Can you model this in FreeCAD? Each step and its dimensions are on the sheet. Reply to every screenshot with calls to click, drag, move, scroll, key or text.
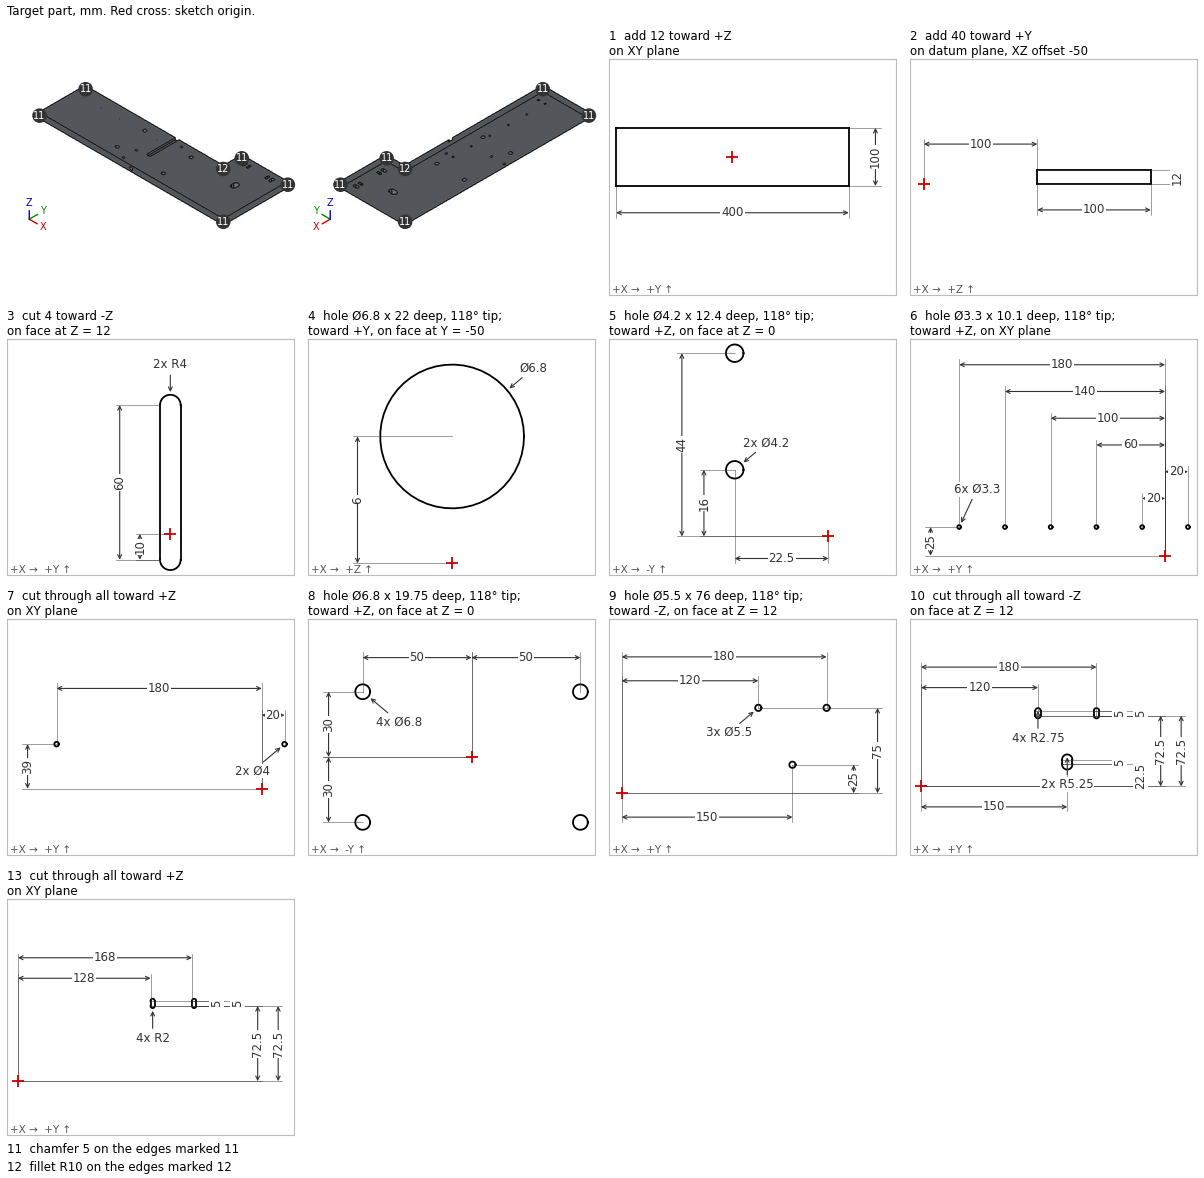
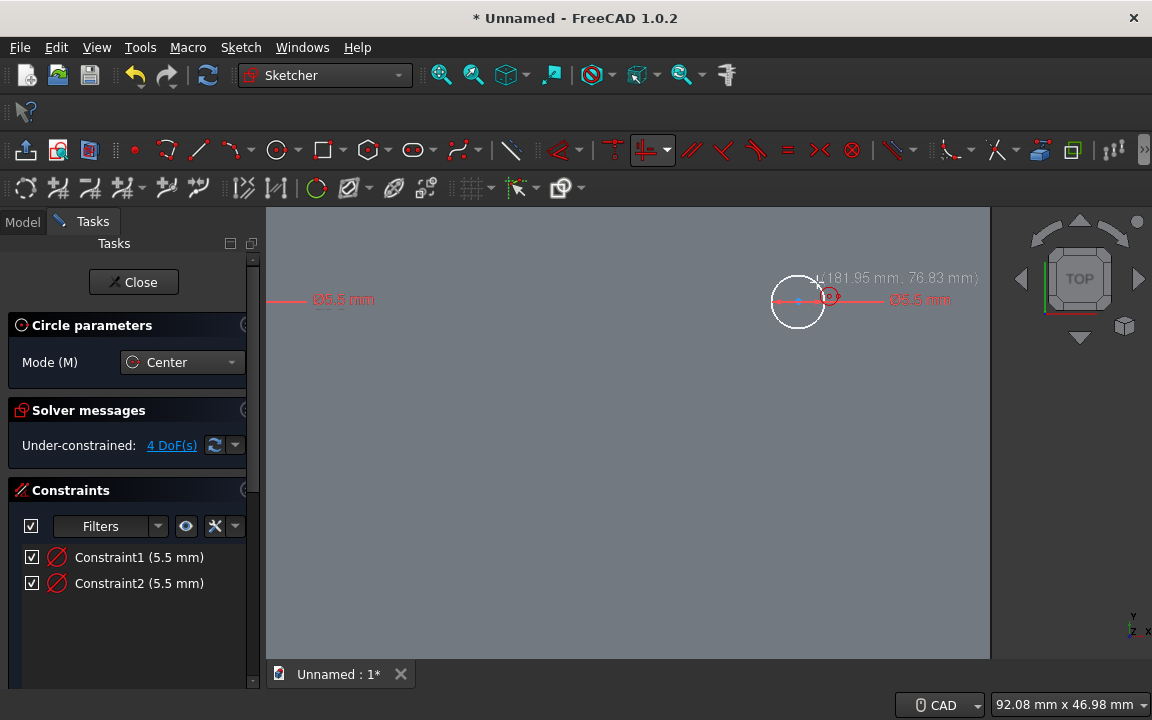
scroll(800, 301, down, 3)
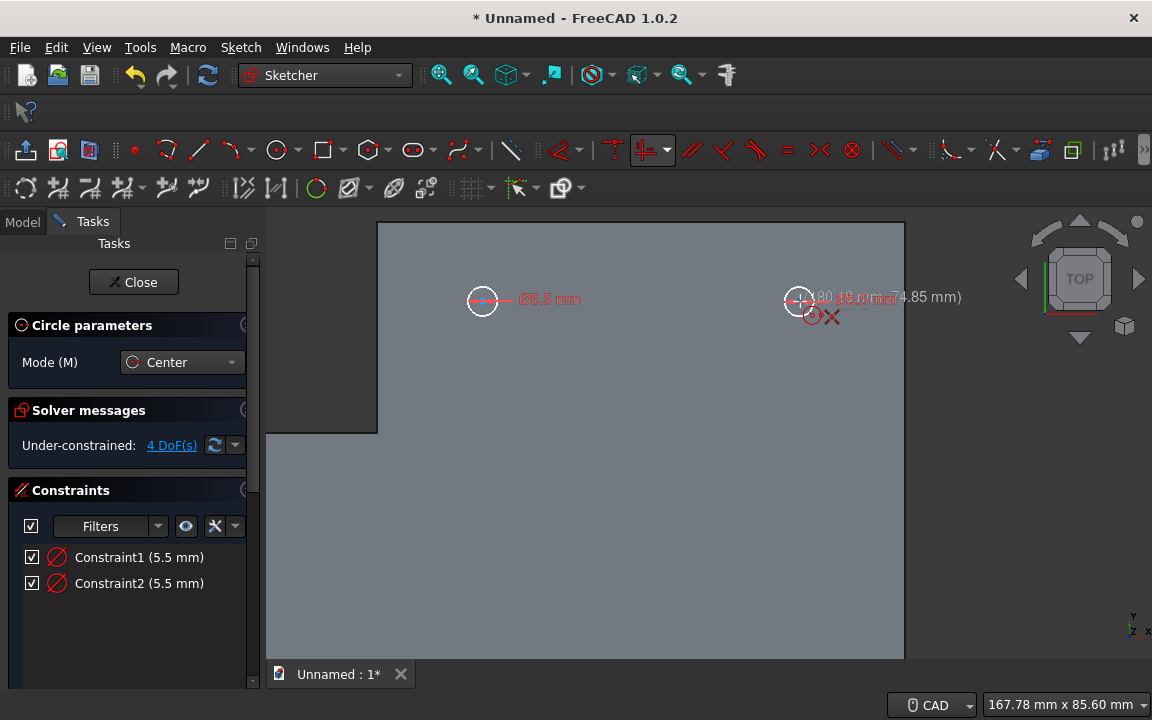
scroll(641, 565, up, 3)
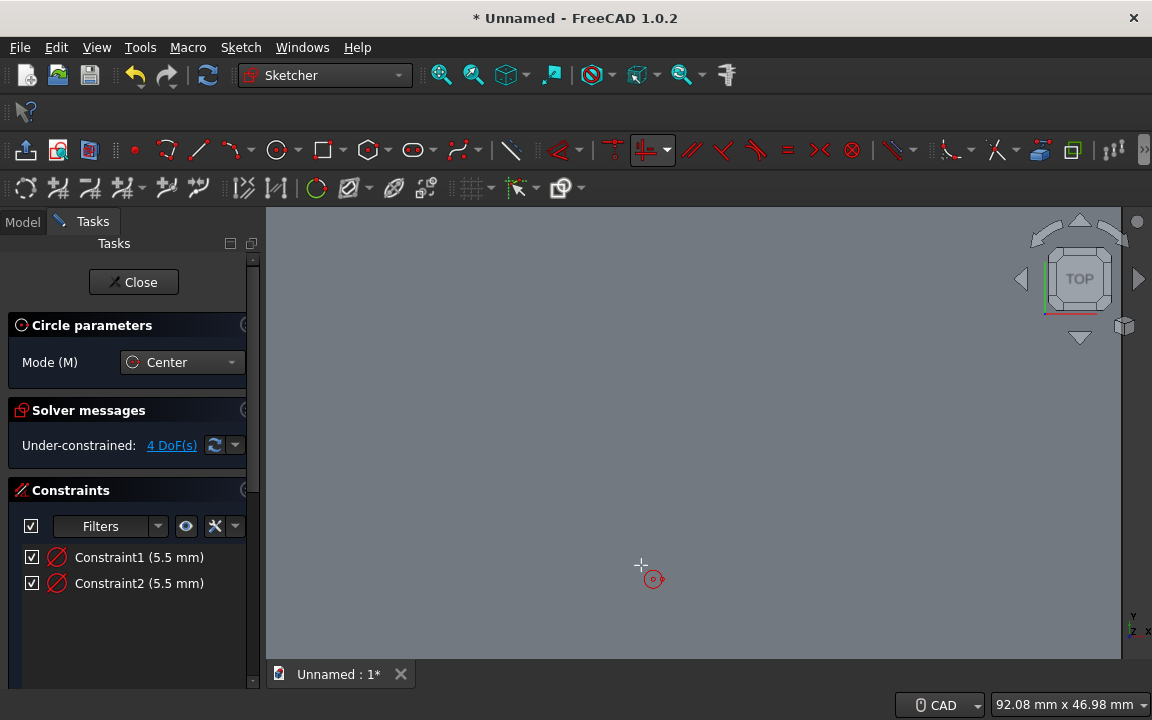
click(640, 564)
move(659, 545)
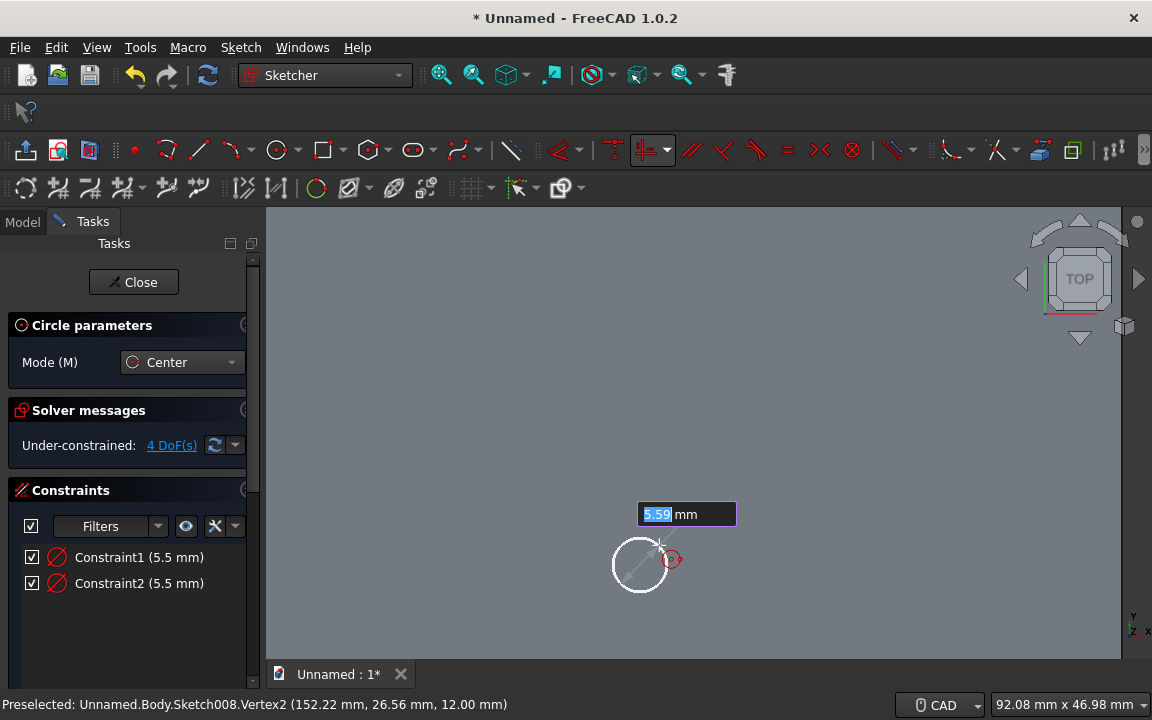
text(5.5)
key(Return)
key(Escape)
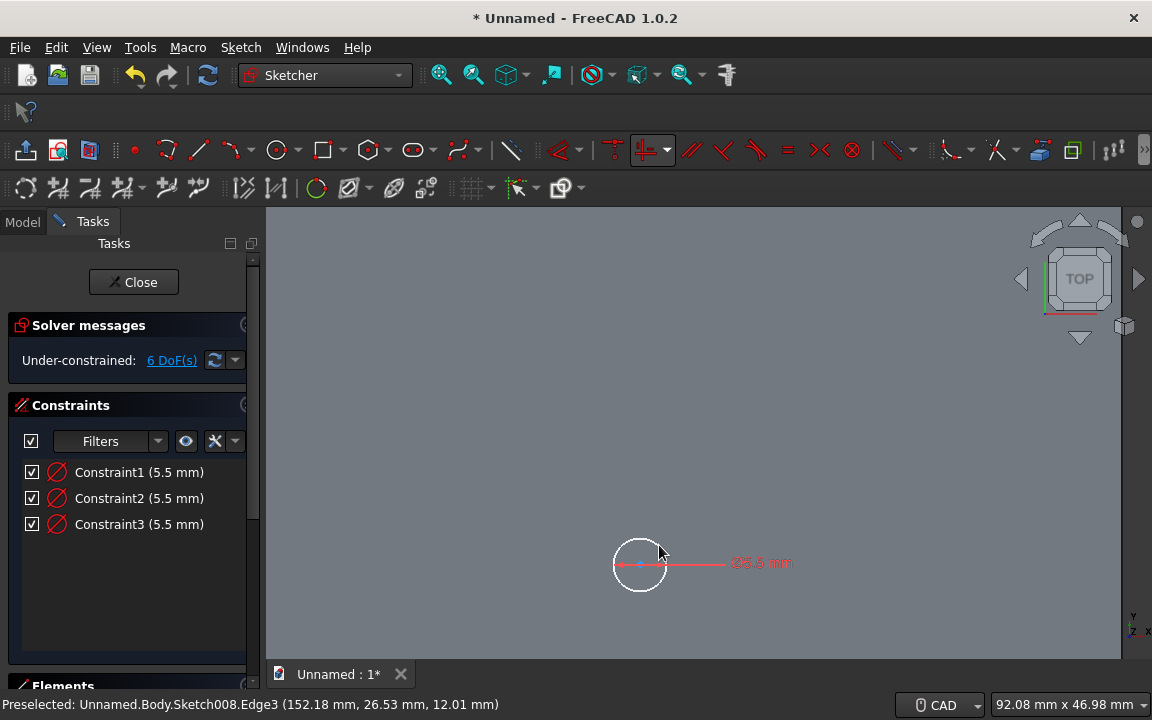
scroll(641, 566, down, 3)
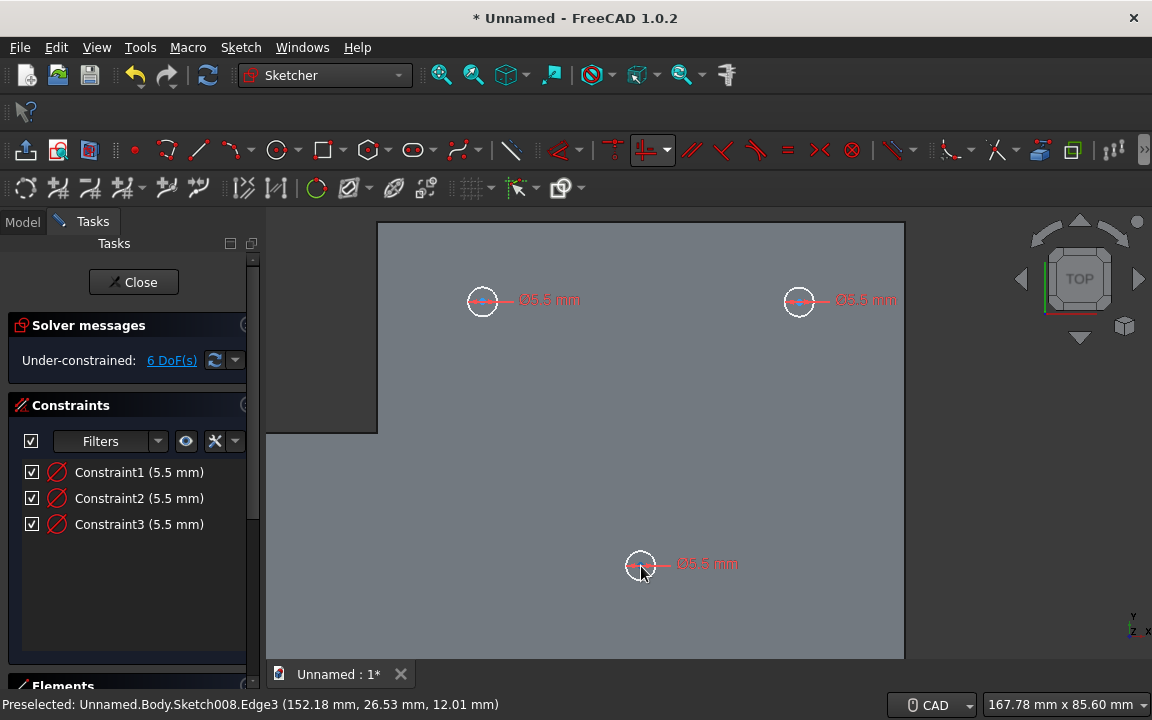
click(483, 302)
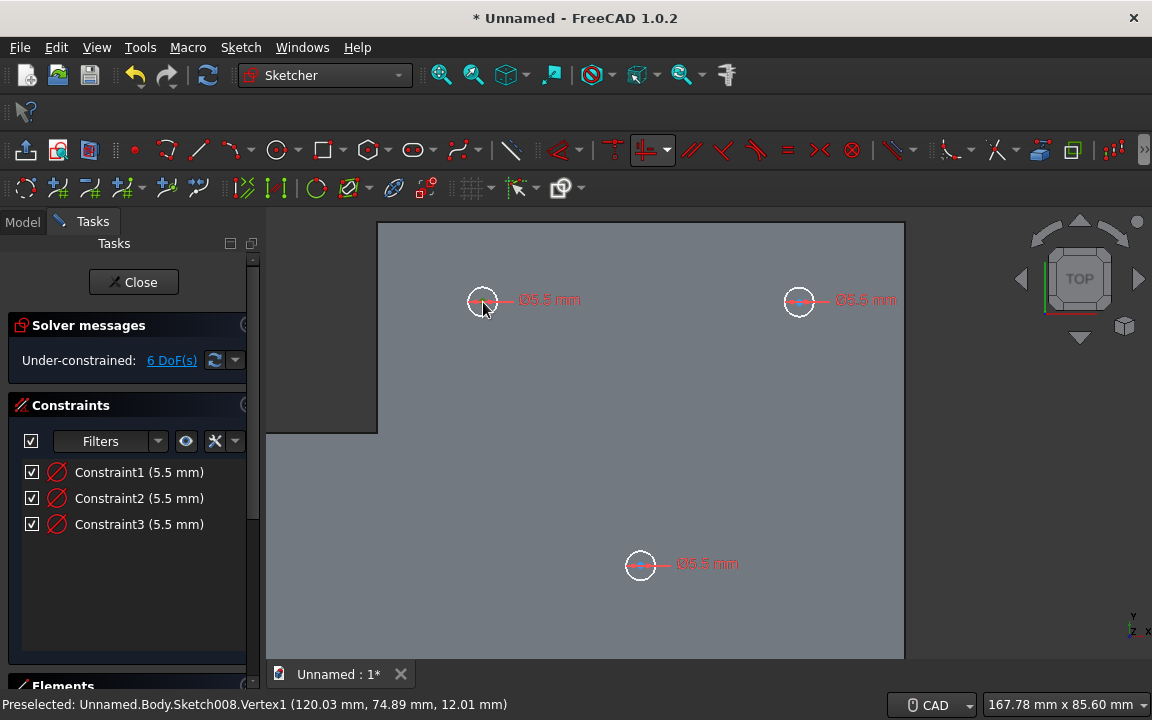
click(799, 302)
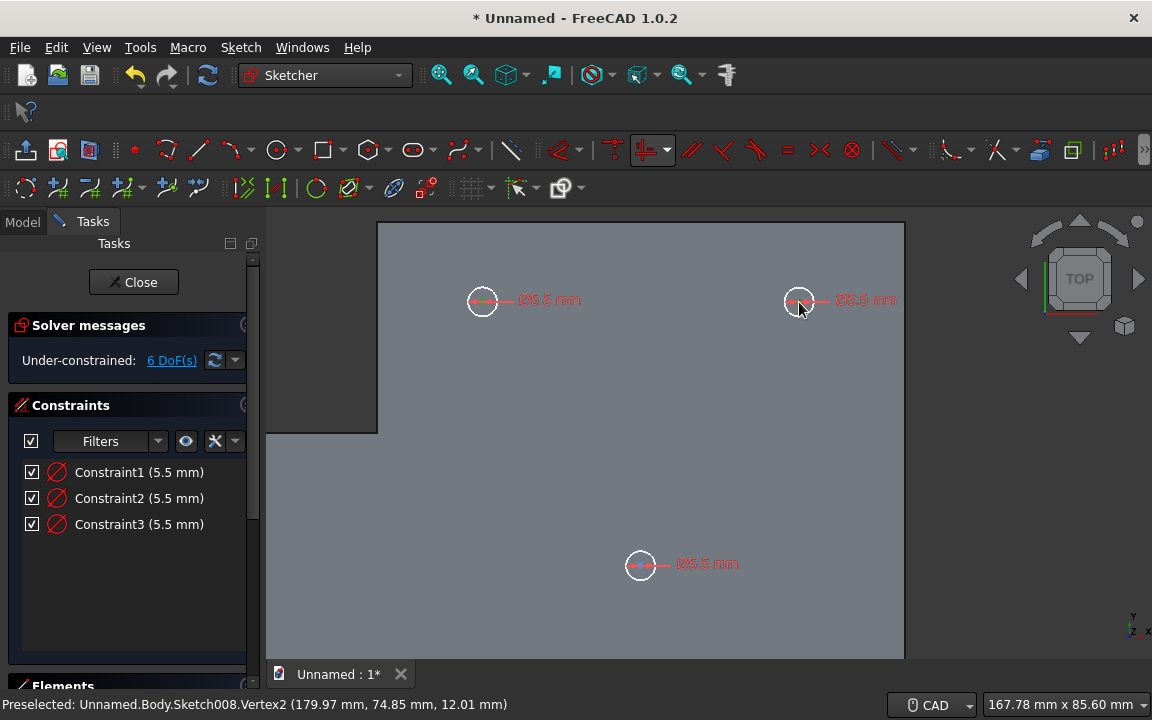
click(670, 150)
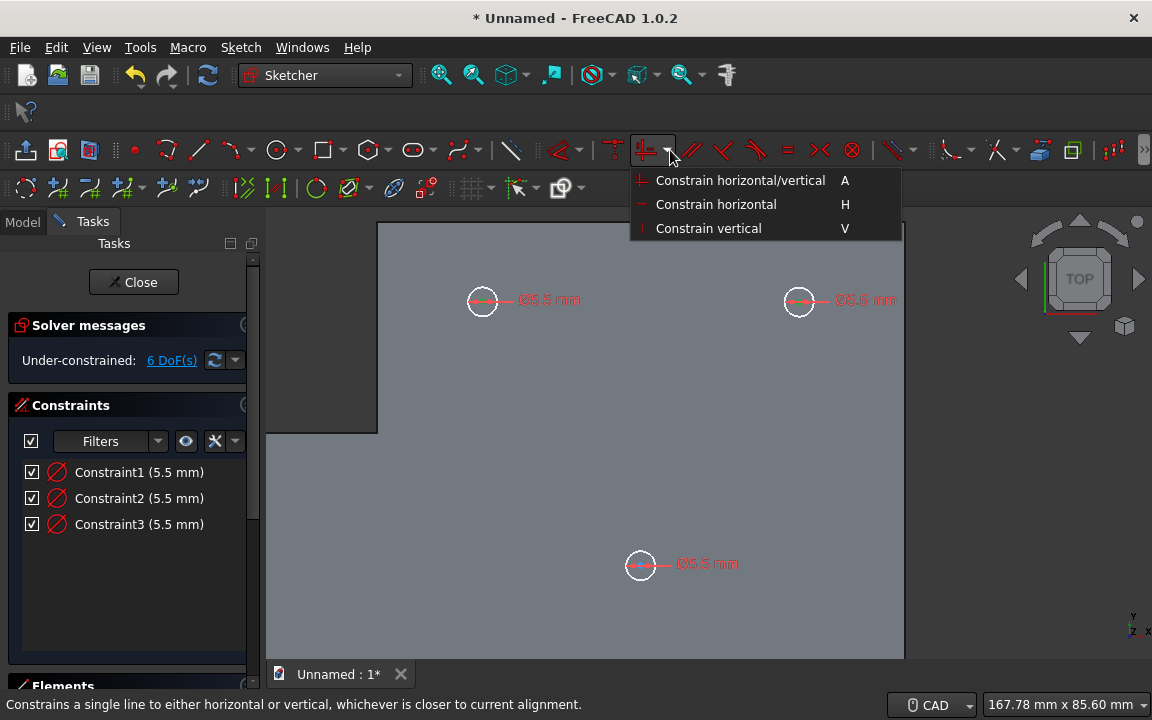
click(766, 204)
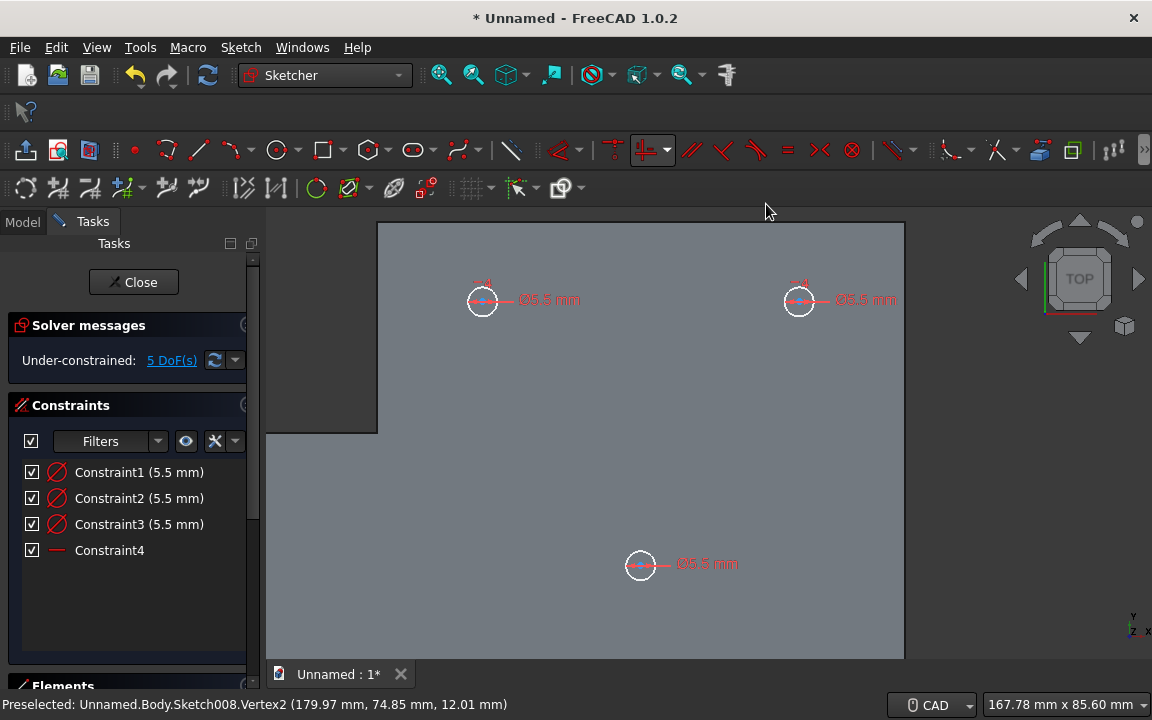
click(558, 150)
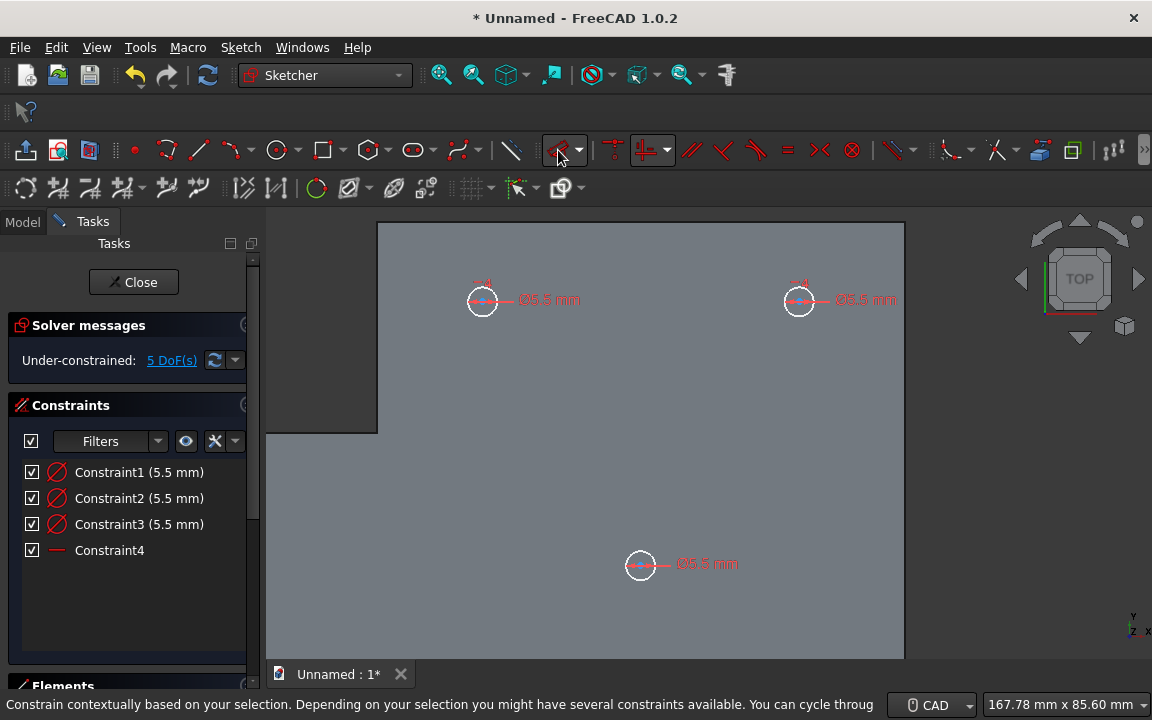
click(483, 302)
click(517, 466)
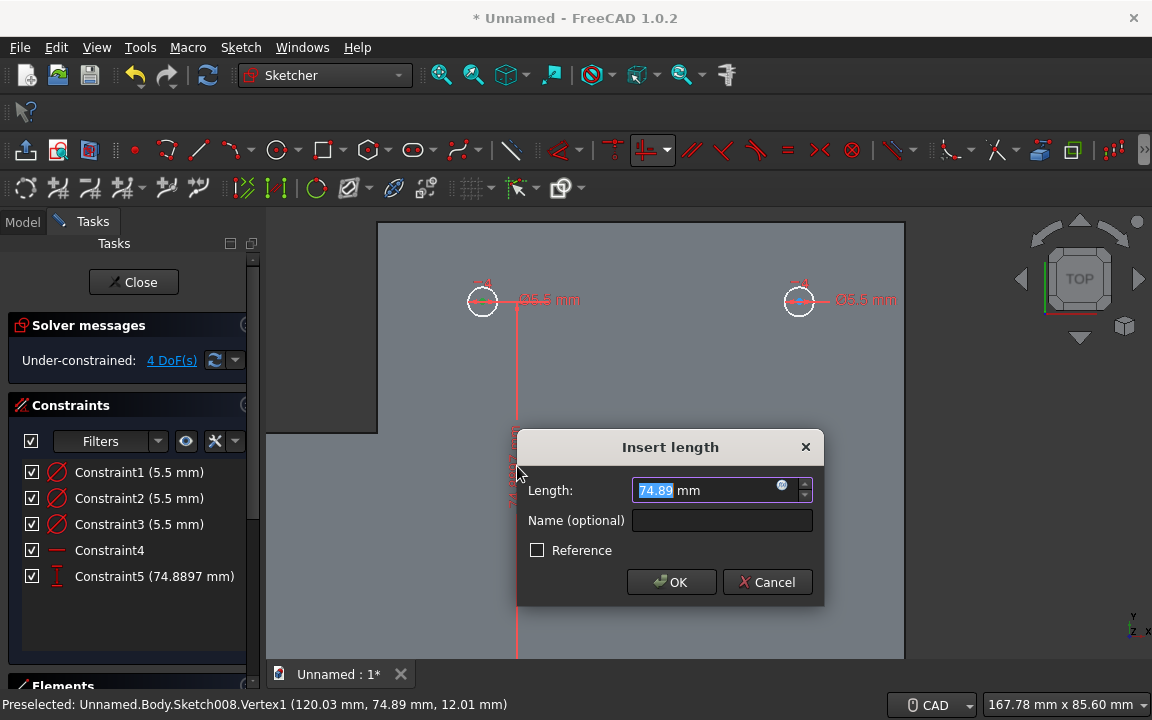
text(75)
key(Return)